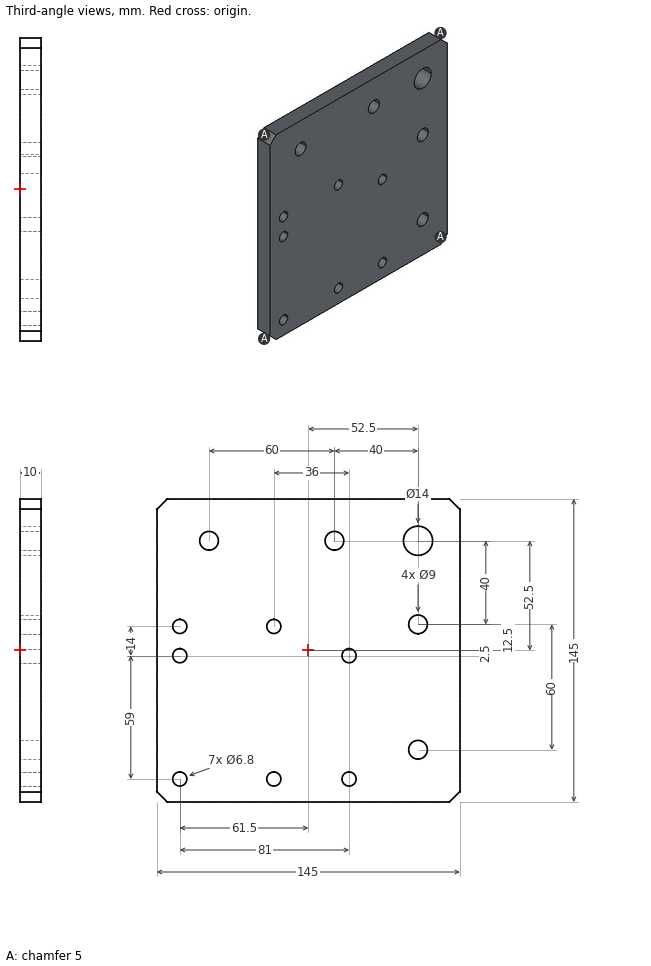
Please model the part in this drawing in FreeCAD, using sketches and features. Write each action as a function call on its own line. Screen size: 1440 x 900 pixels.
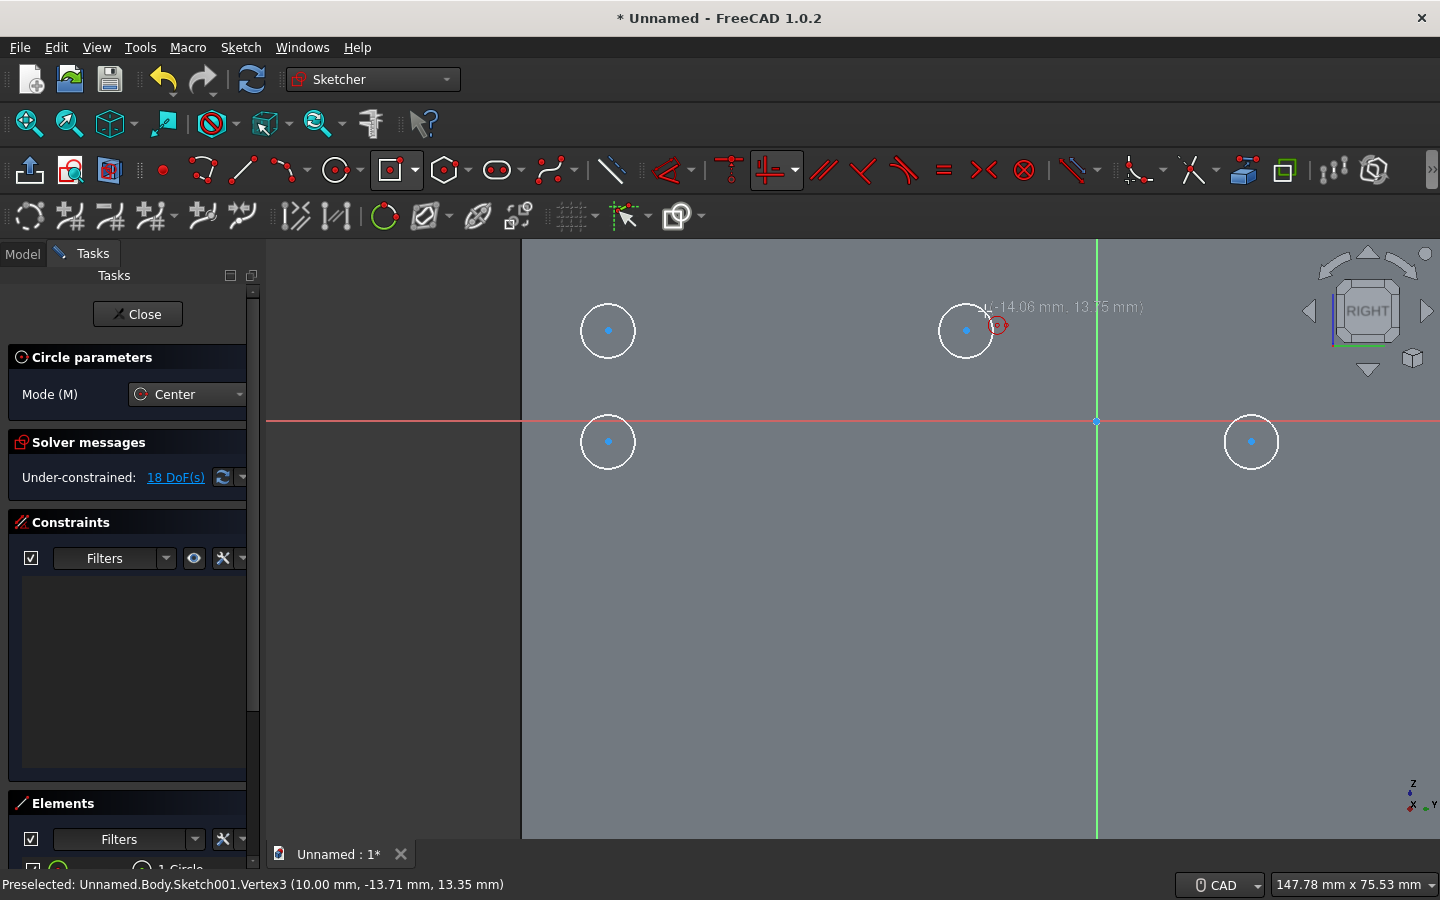
scroll(608, 441, down, 3)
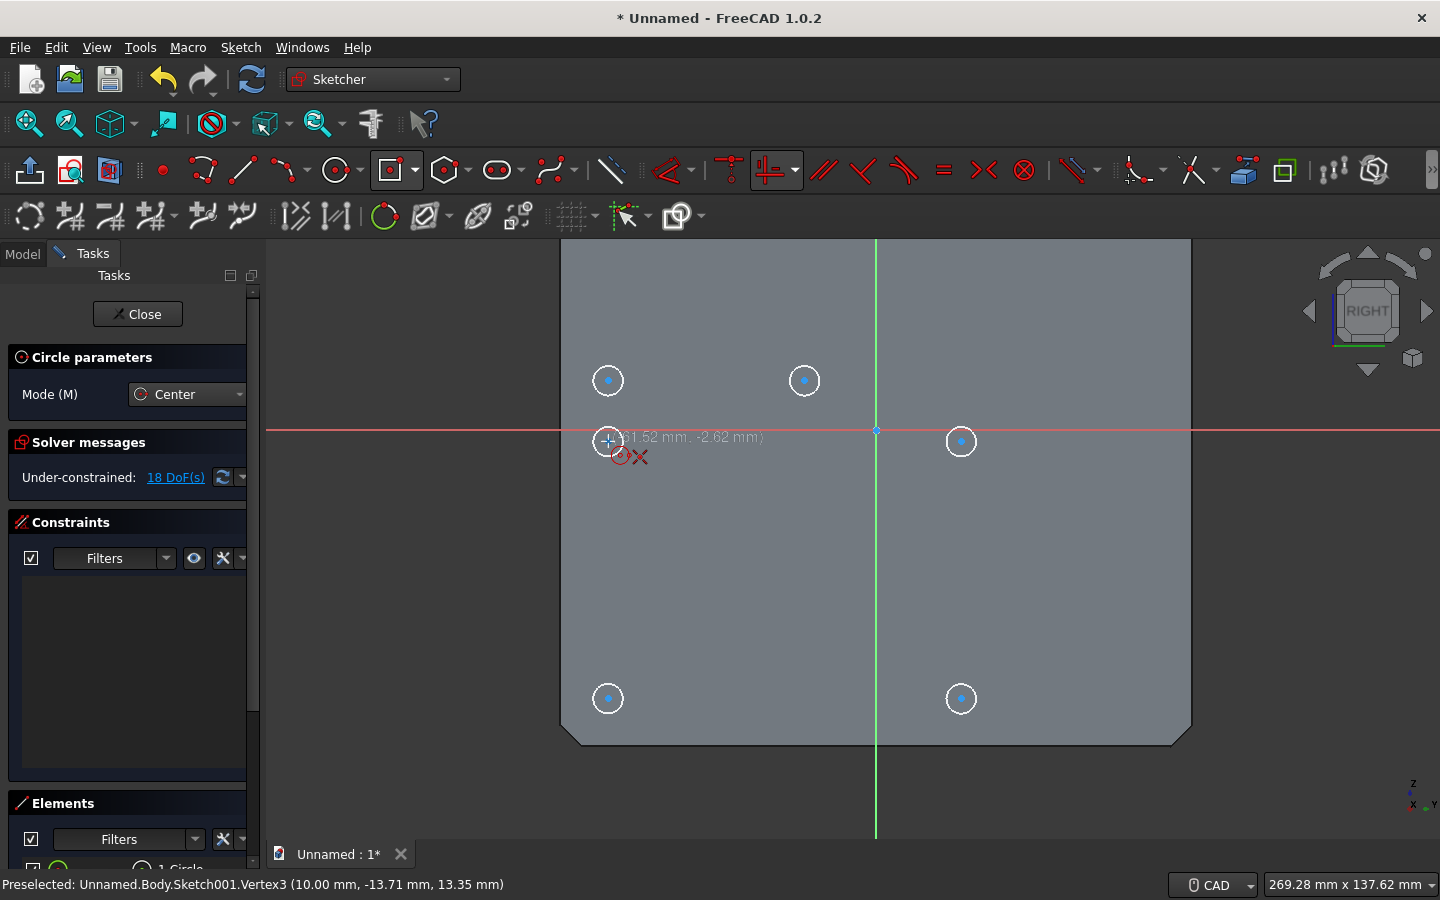
scroll(804, 698, up, 3)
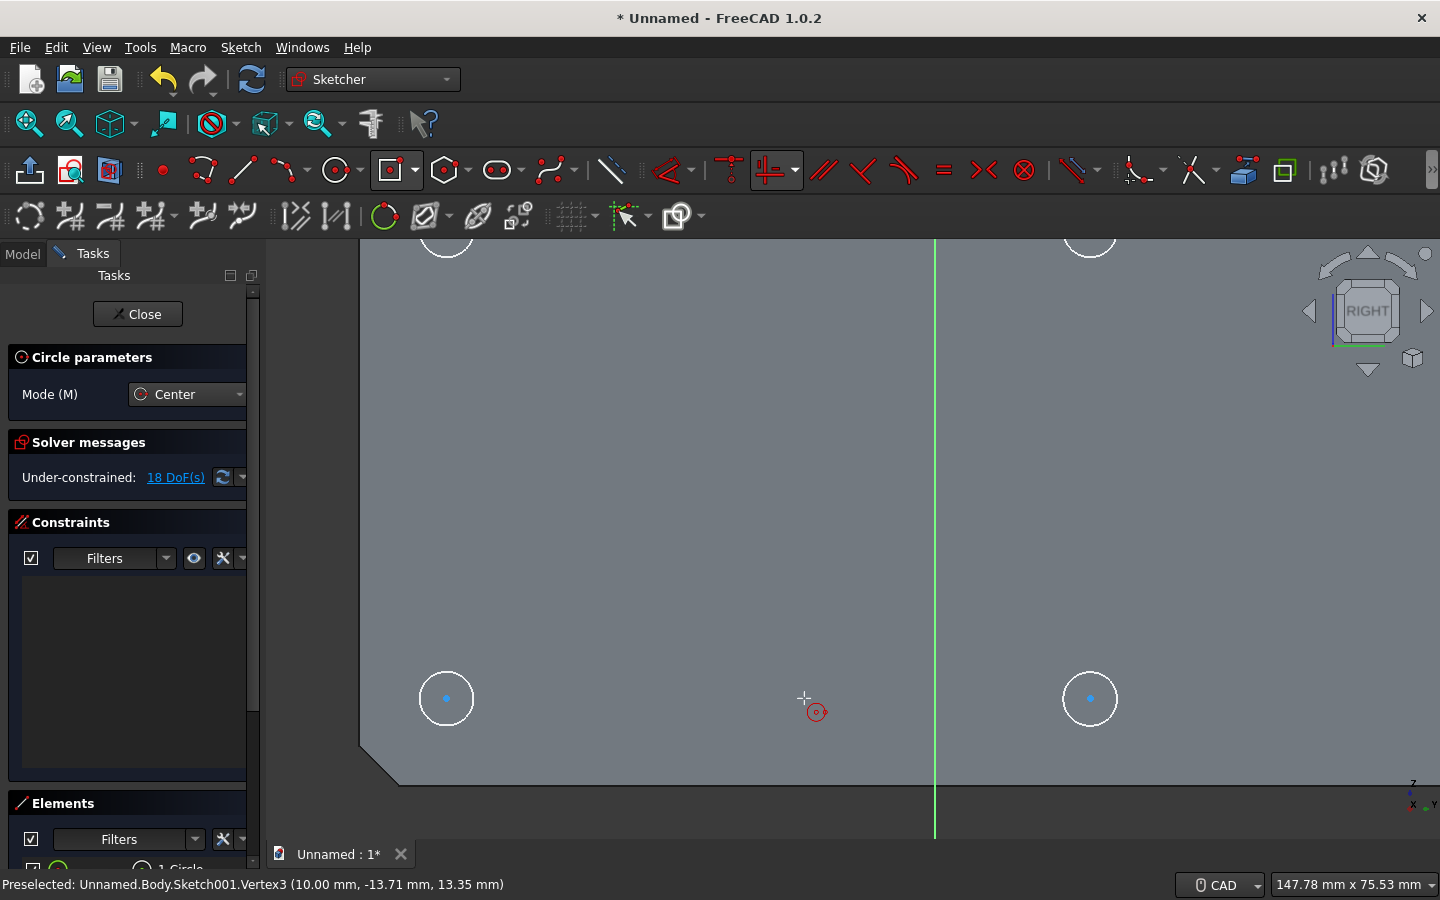
click(804, 698)
click(823, 679)
key(Escape)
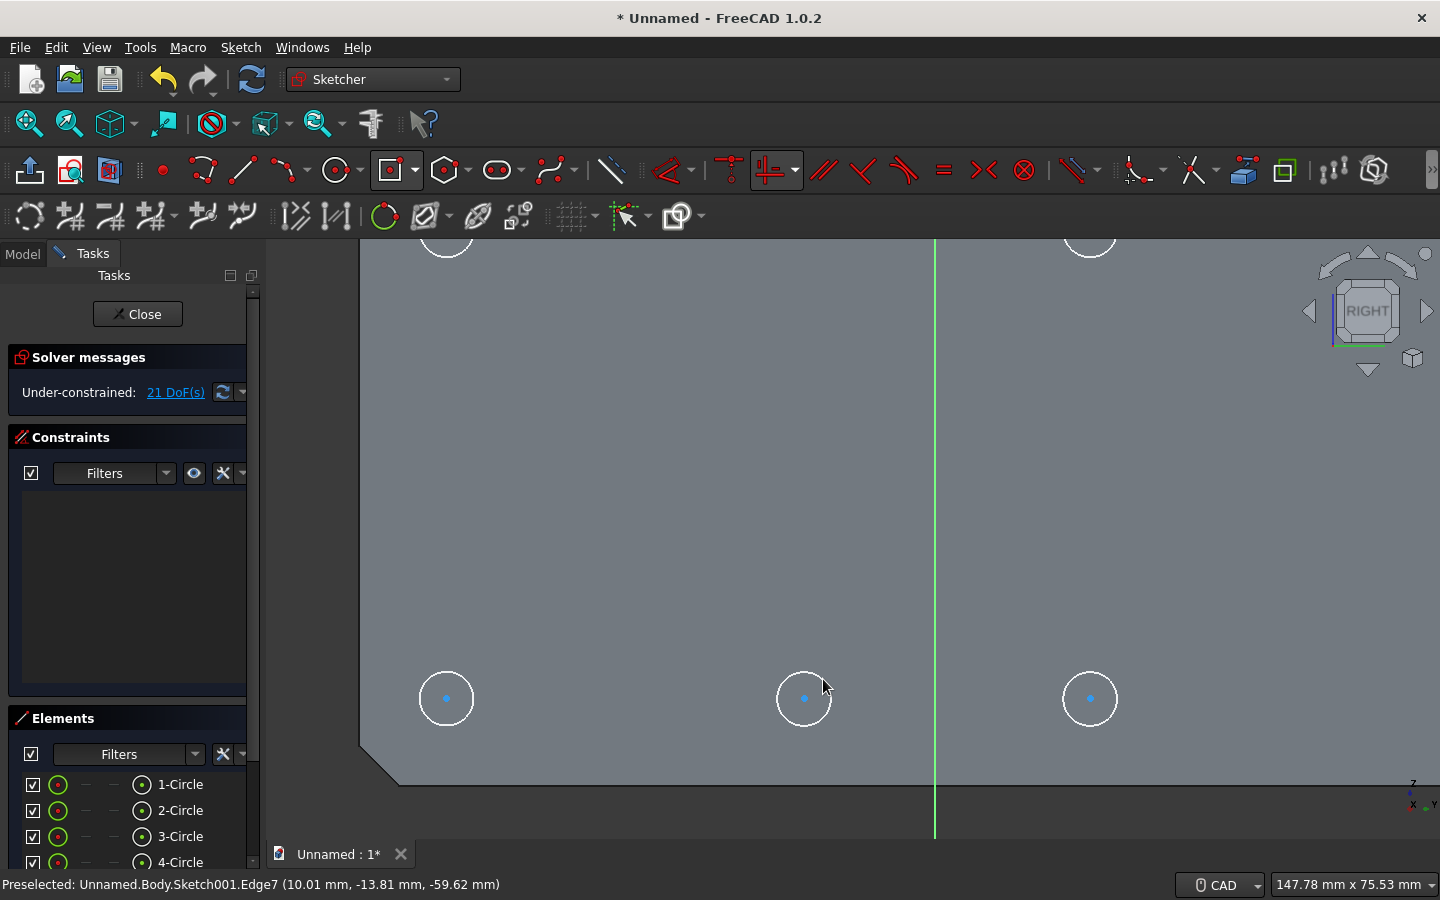
click(465, 680)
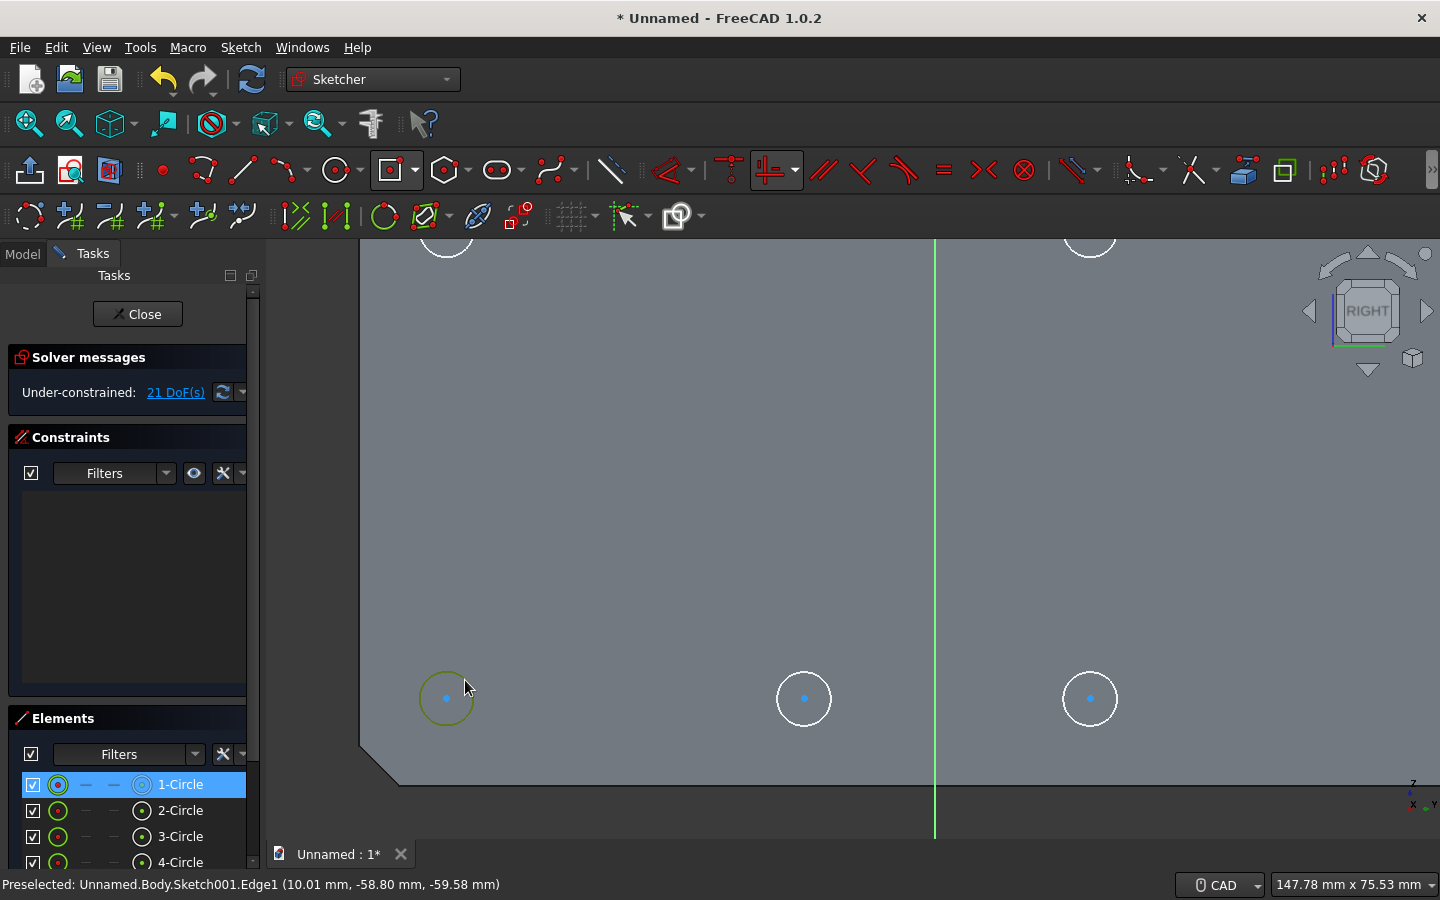
scroll(804, 698, down, 3)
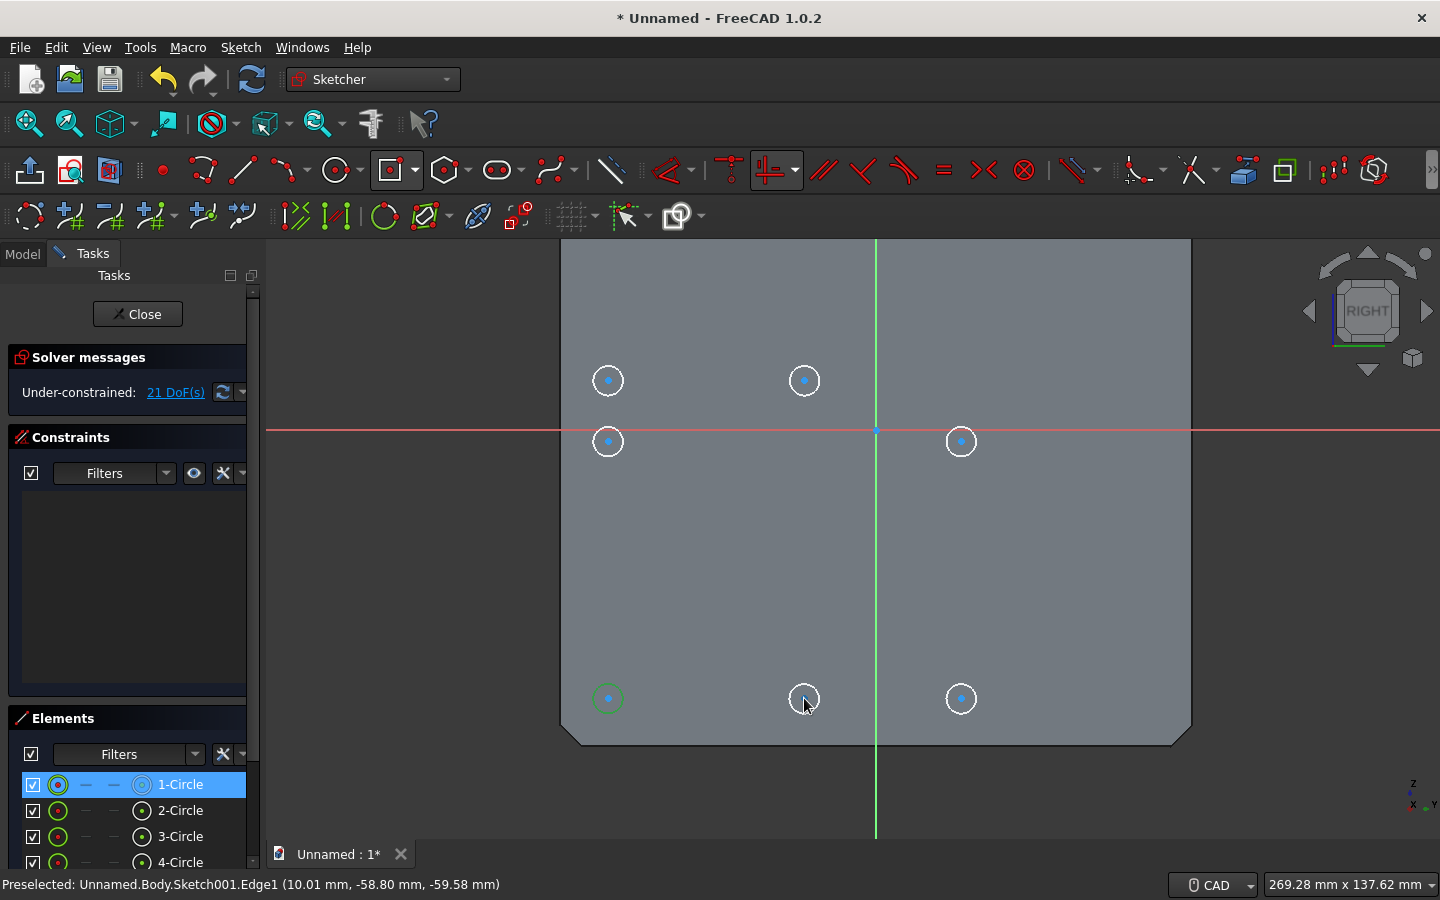
click(972, 431)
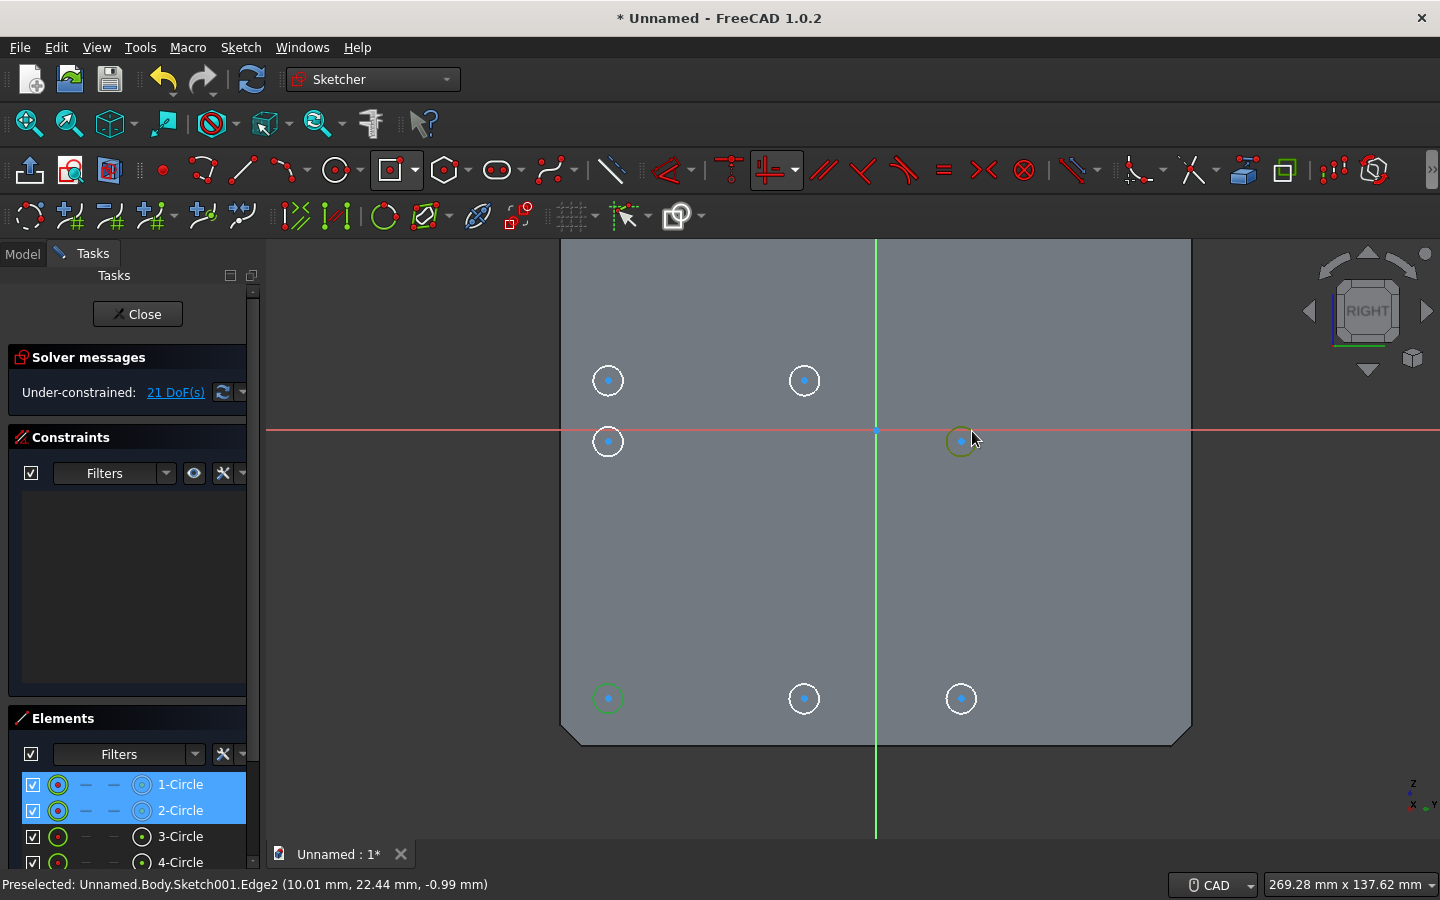
click(972, 688)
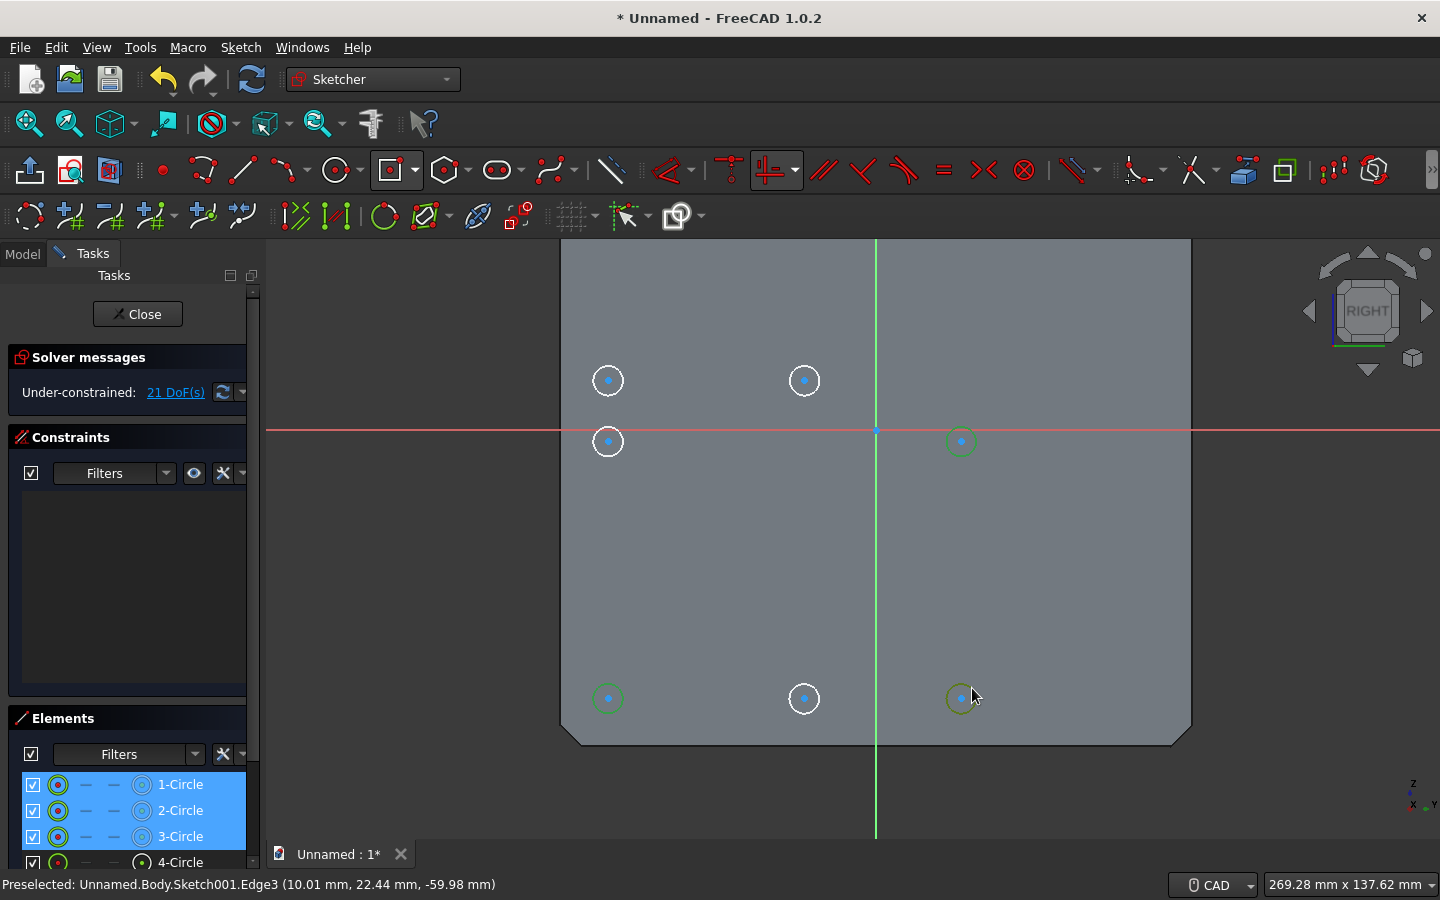
click(619, 431)